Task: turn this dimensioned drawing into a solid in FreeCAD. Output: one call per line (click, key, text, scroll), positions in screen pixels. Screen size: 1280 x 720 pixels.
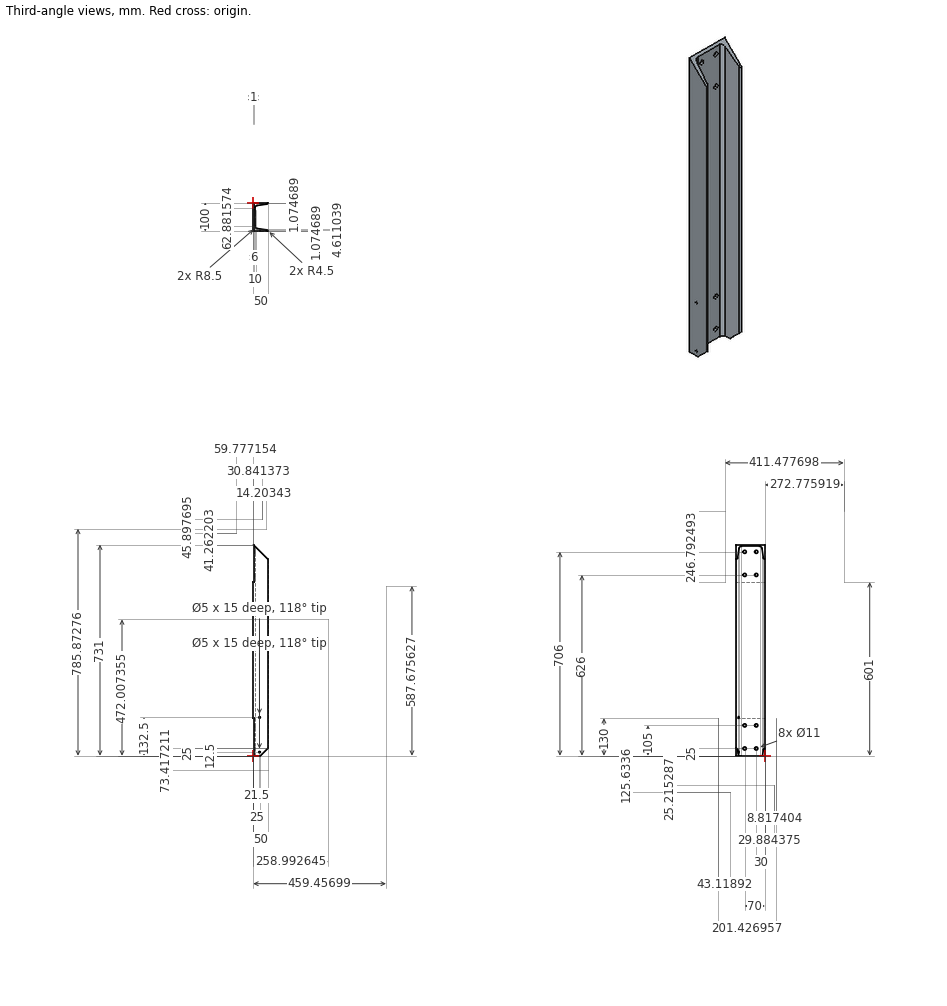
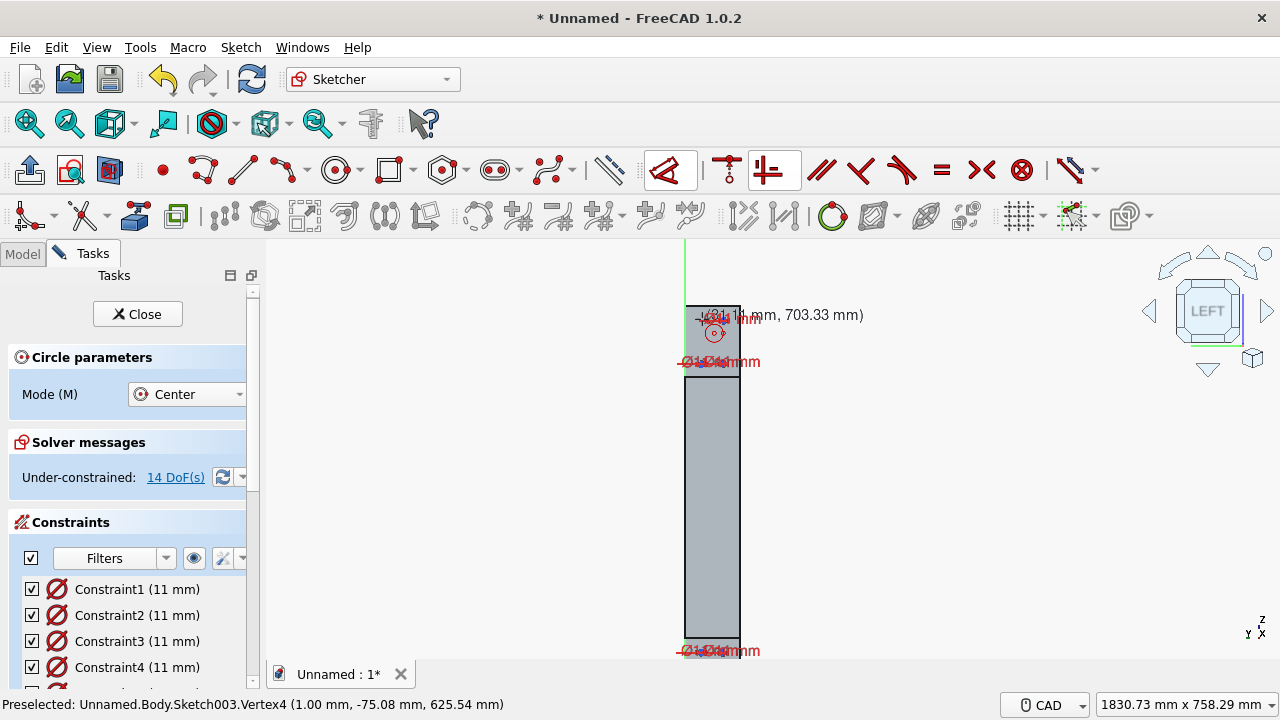
click(701, 319)
move(703, 317)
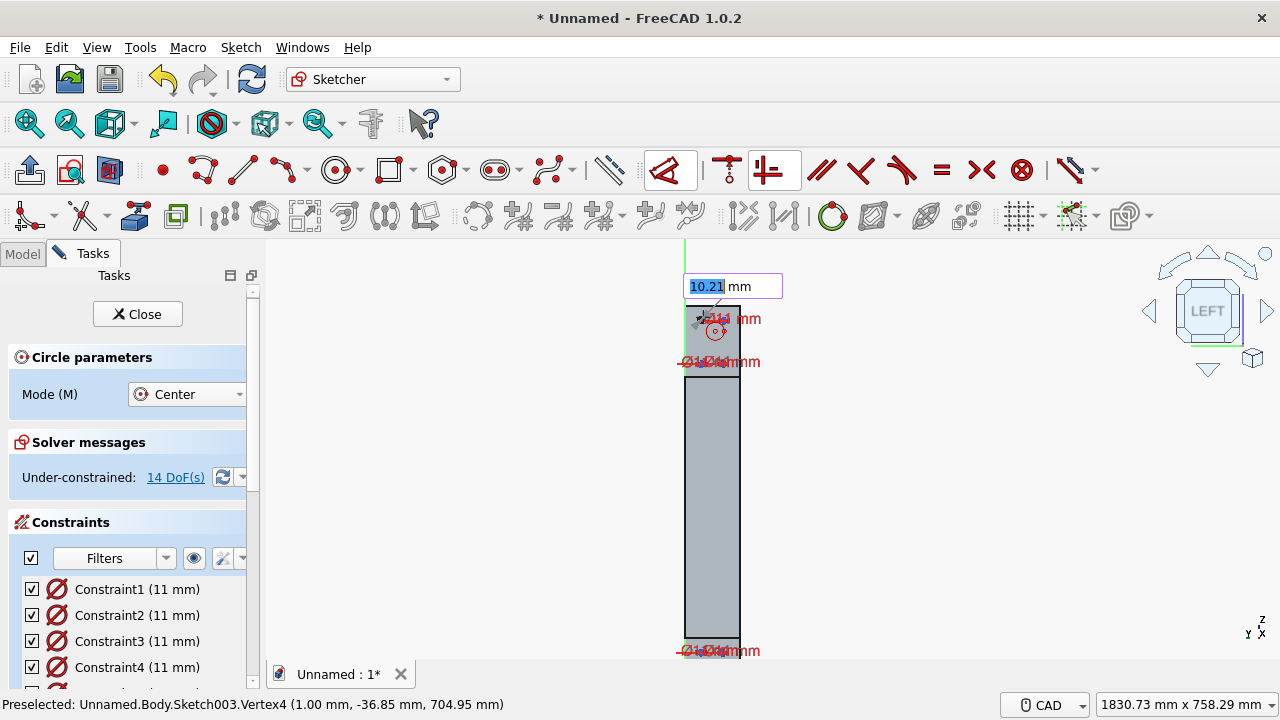
text(11)
key(Return)
key(Escape)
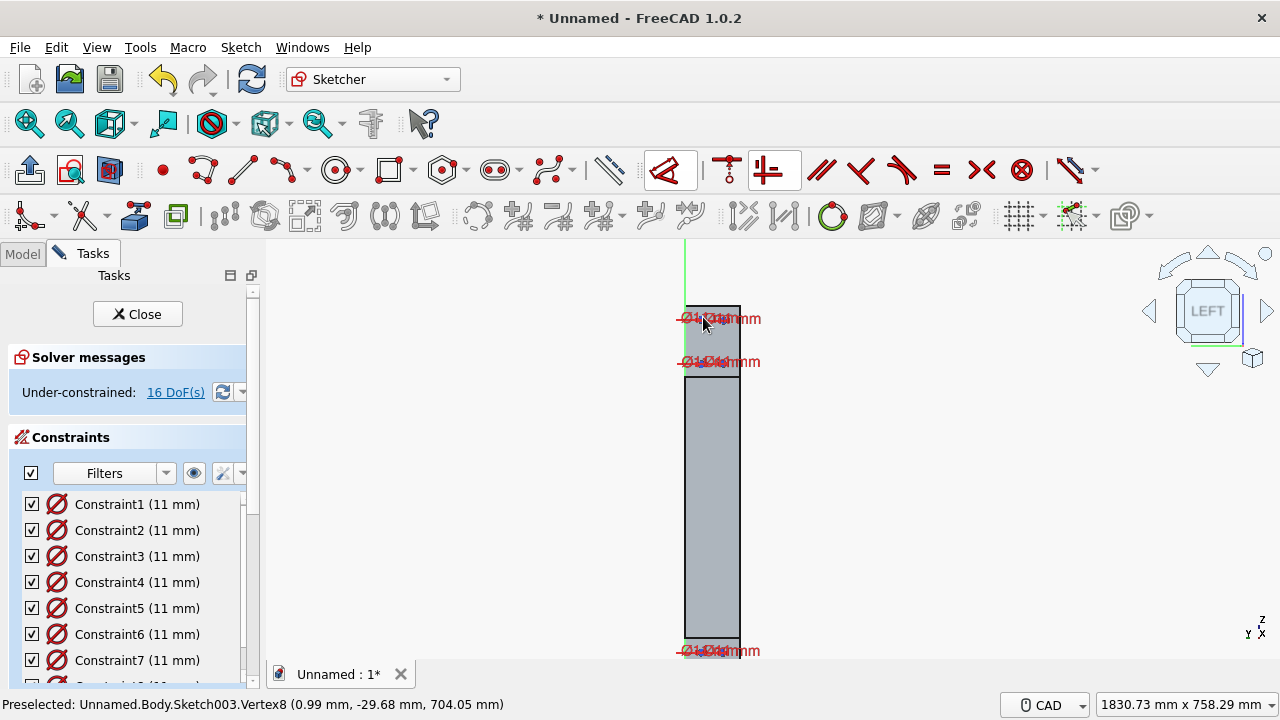
scroll(703, 319, down, 2)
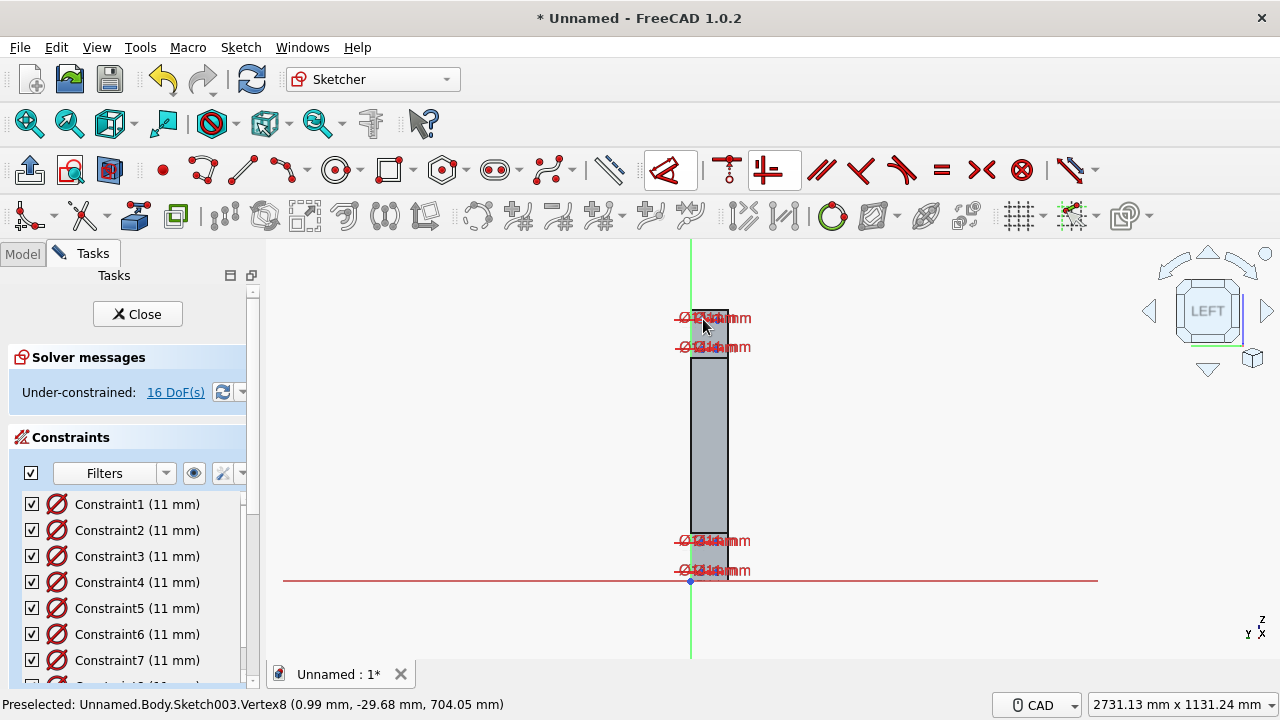
scroll(702, 572, up, 7)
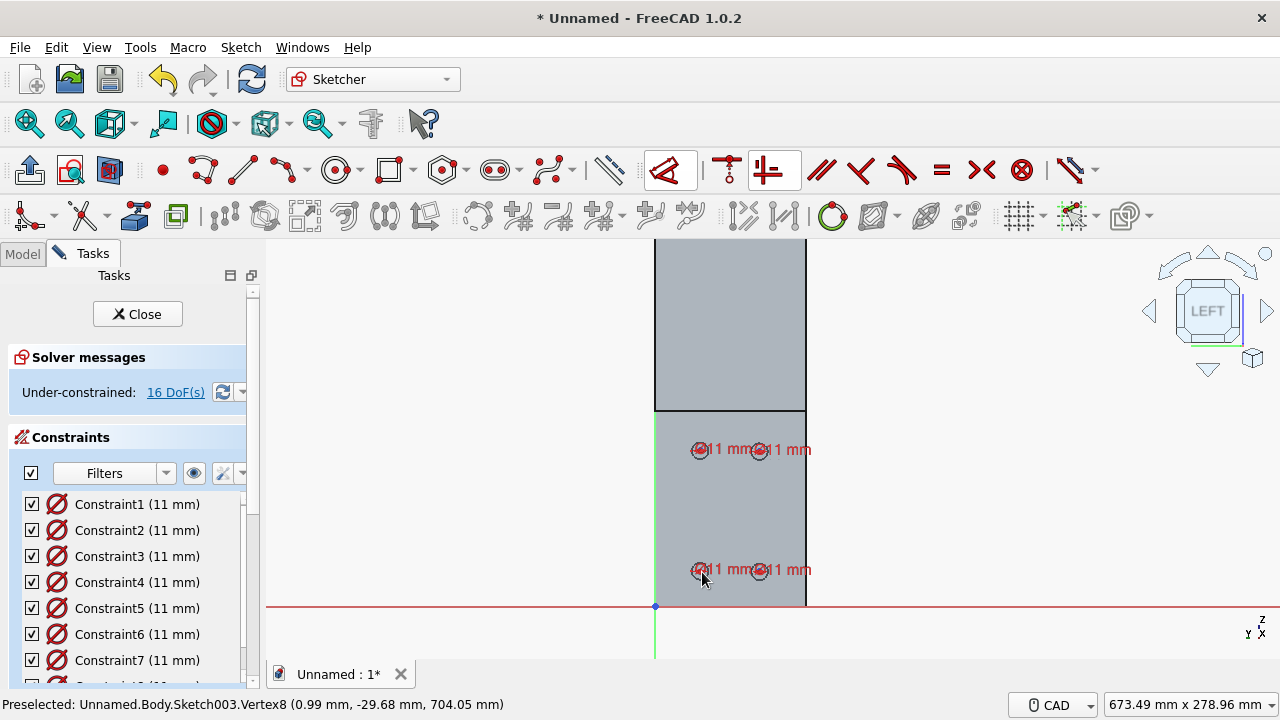
click(700, 571)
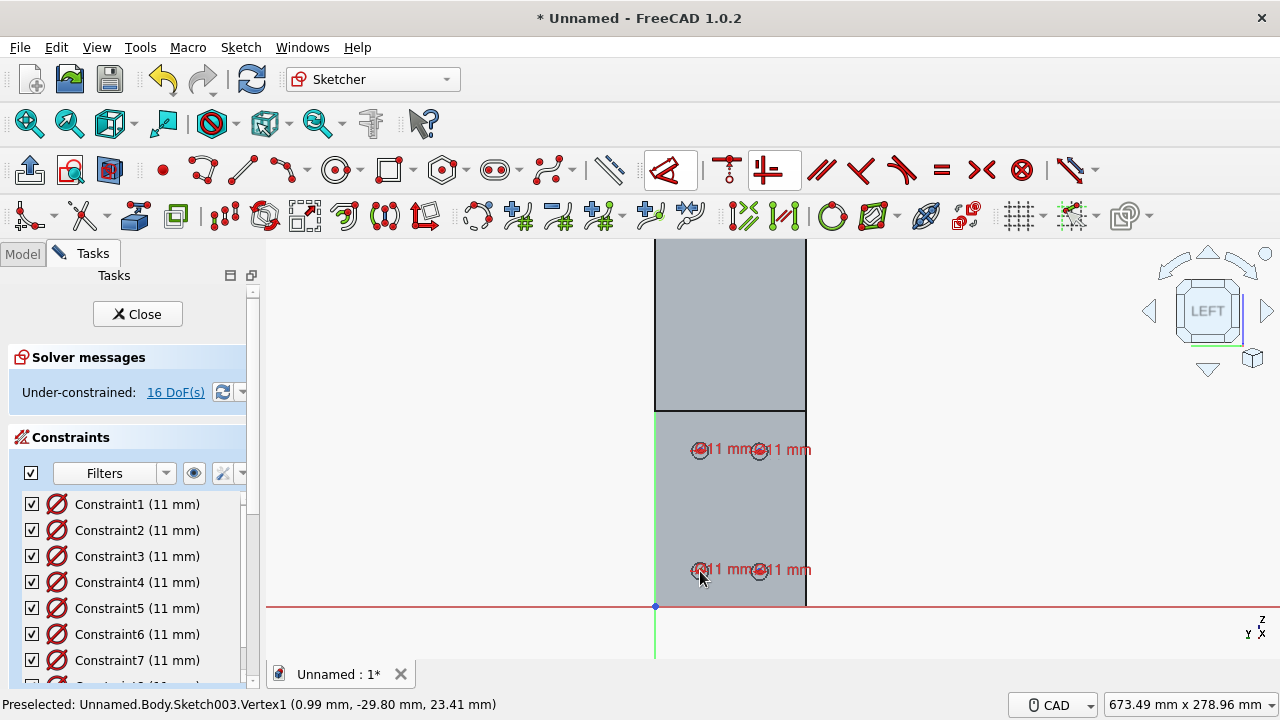
key(l)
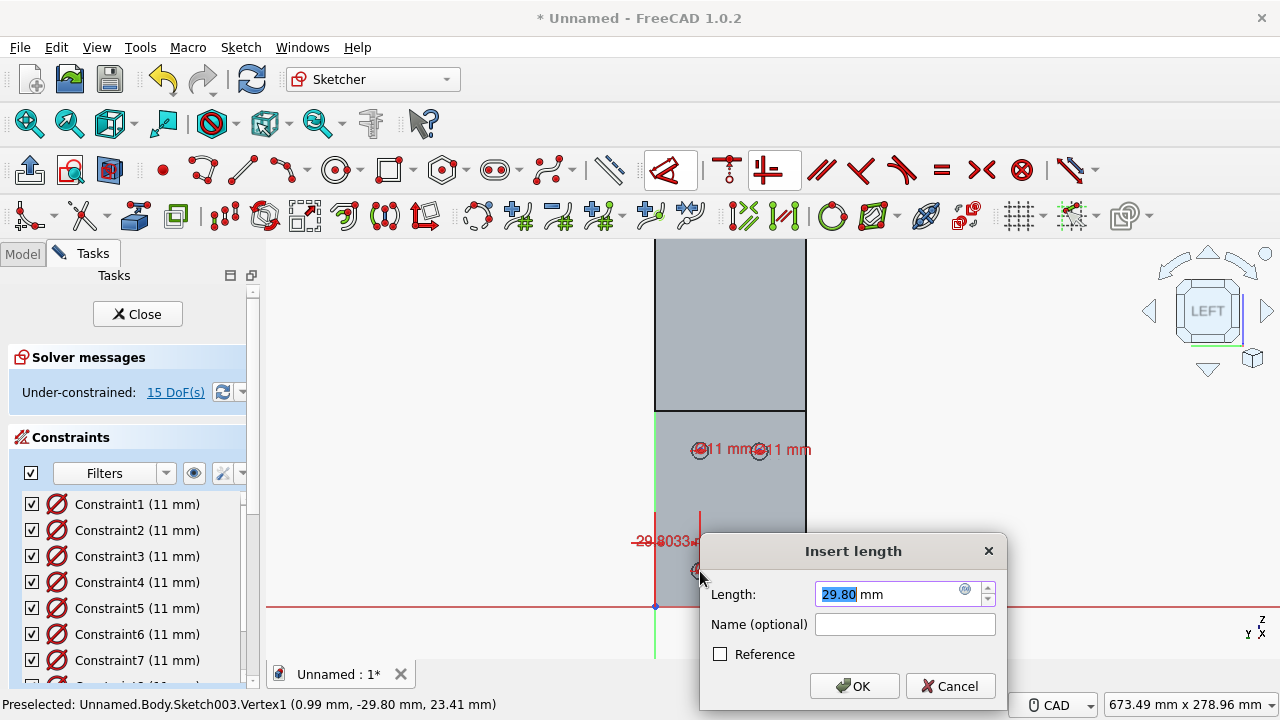
text(30)
key(Return)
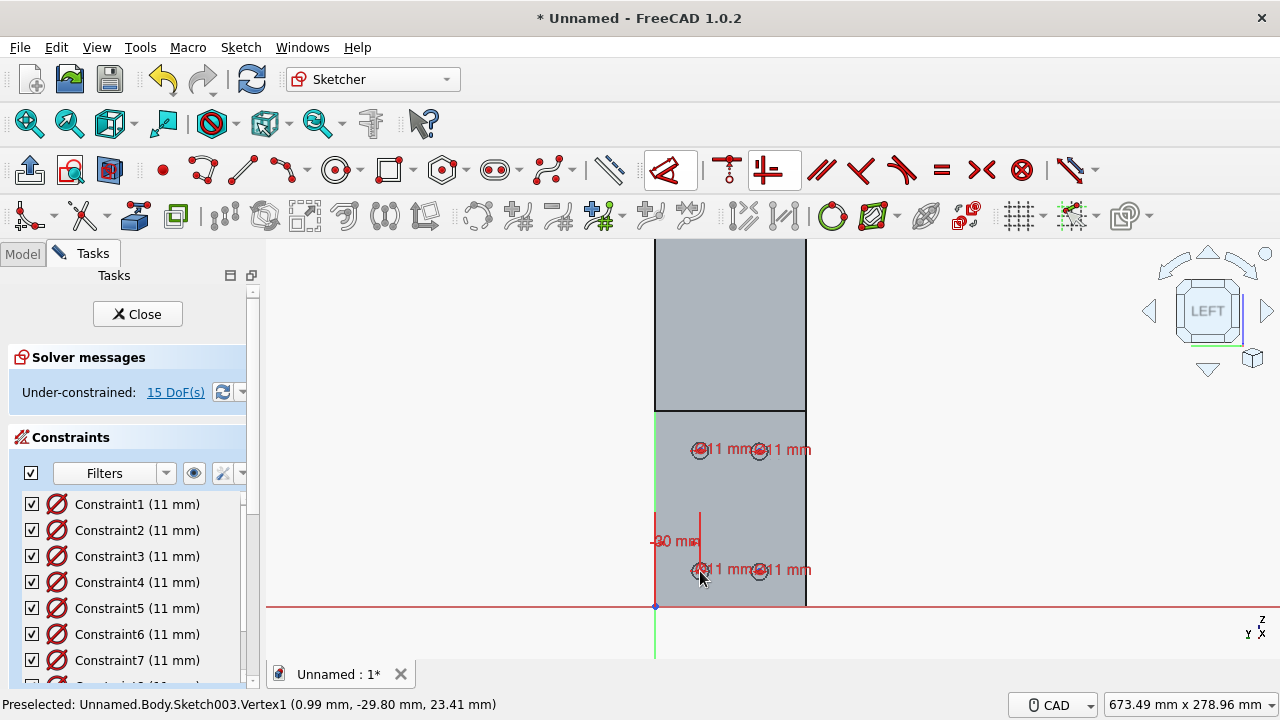
click(700, 571)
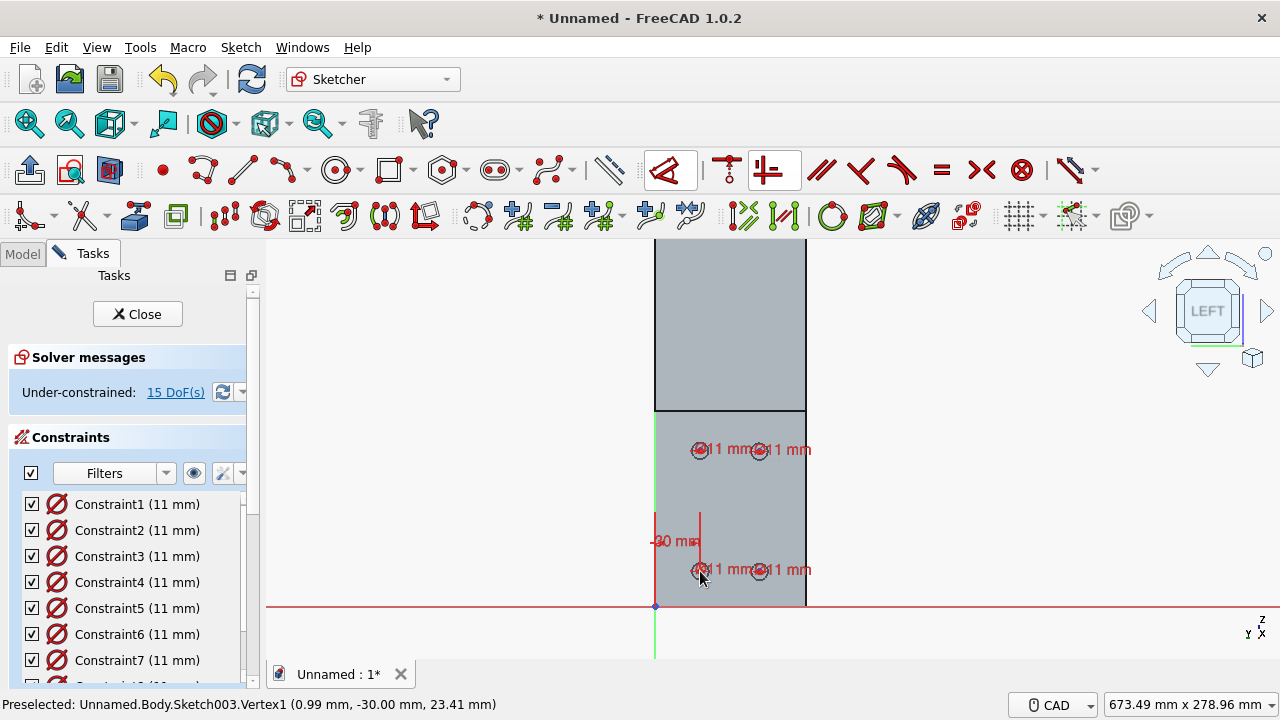
key(i)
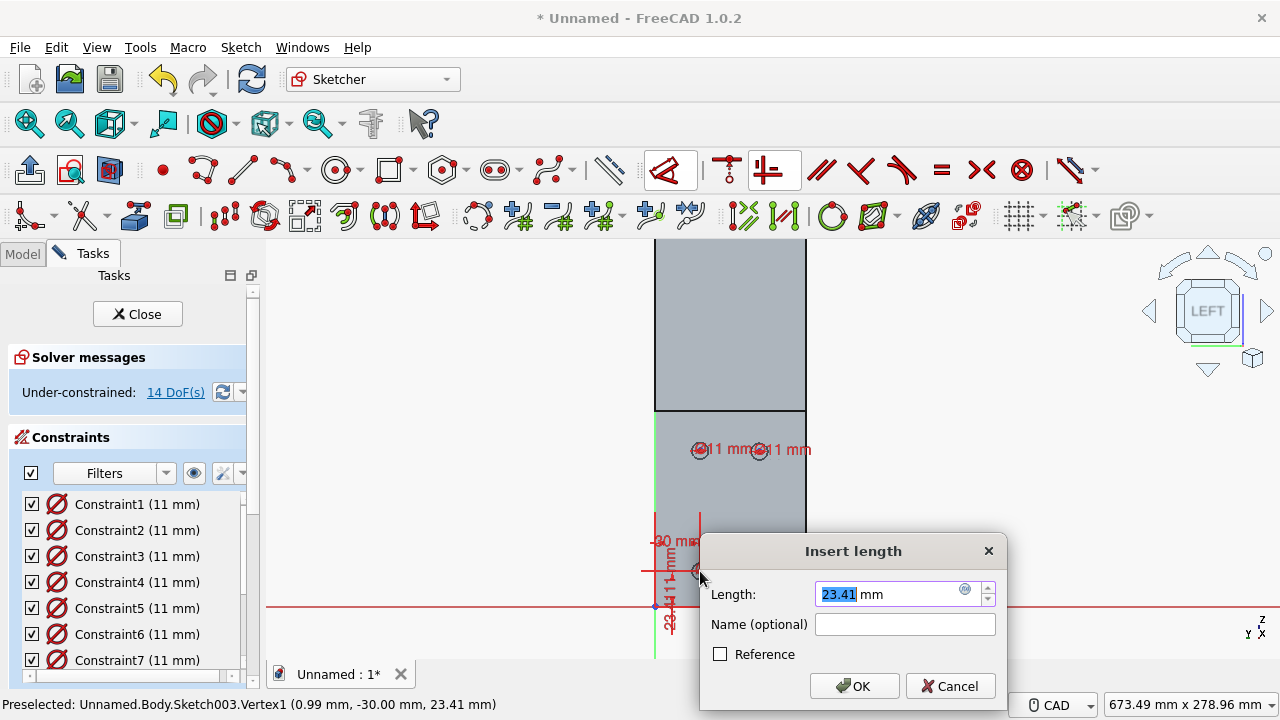
text(25)
key(Return)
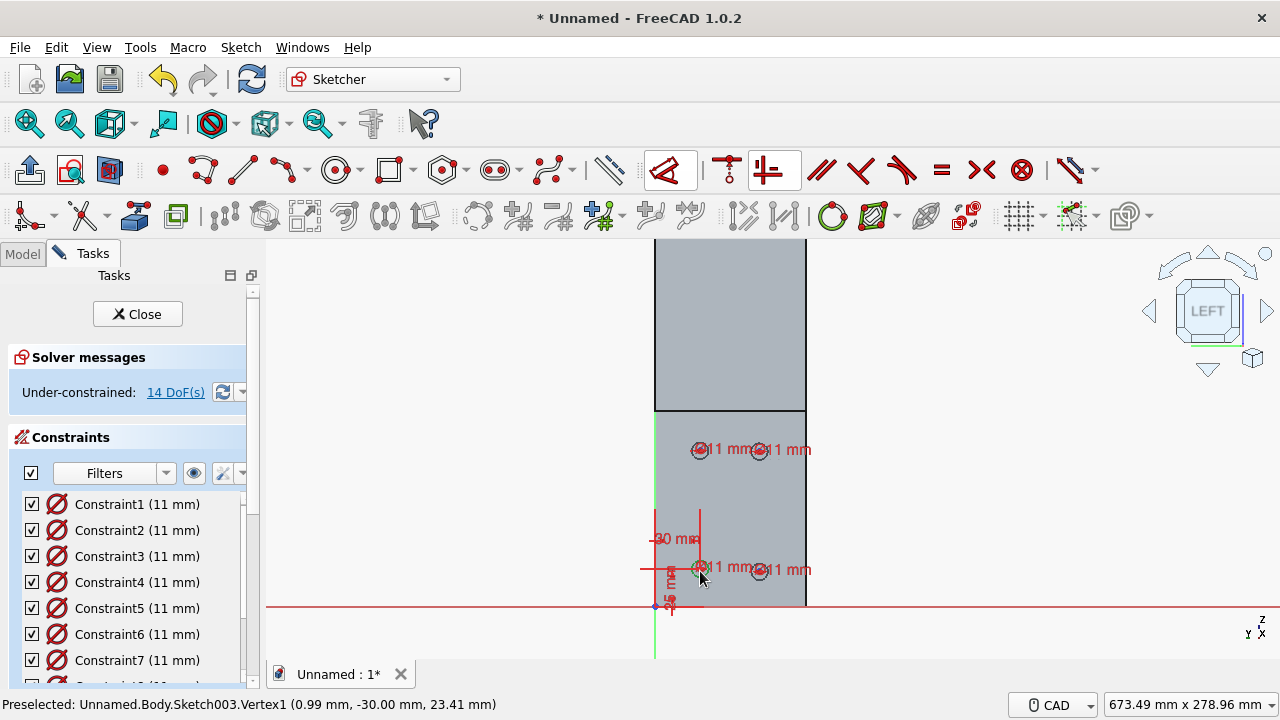
click(700, 451)